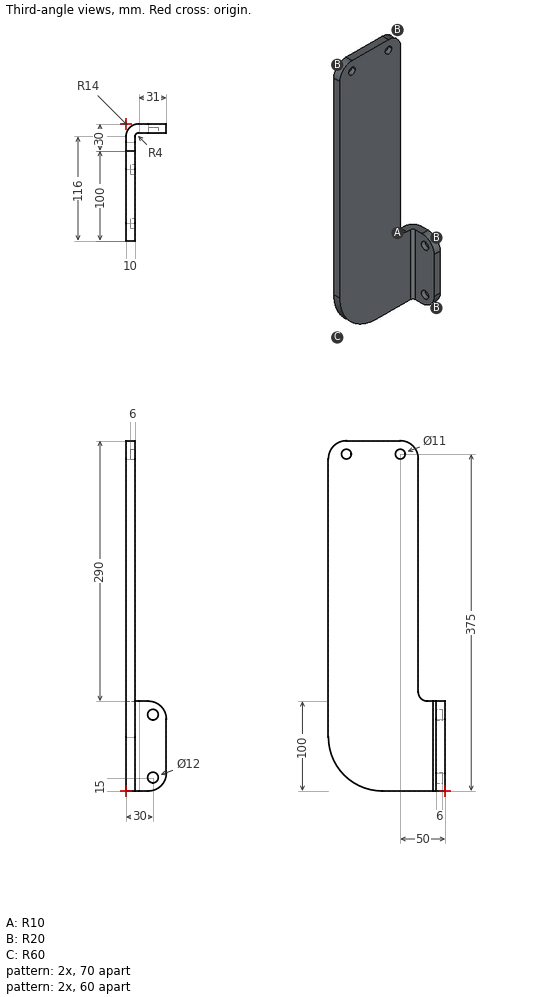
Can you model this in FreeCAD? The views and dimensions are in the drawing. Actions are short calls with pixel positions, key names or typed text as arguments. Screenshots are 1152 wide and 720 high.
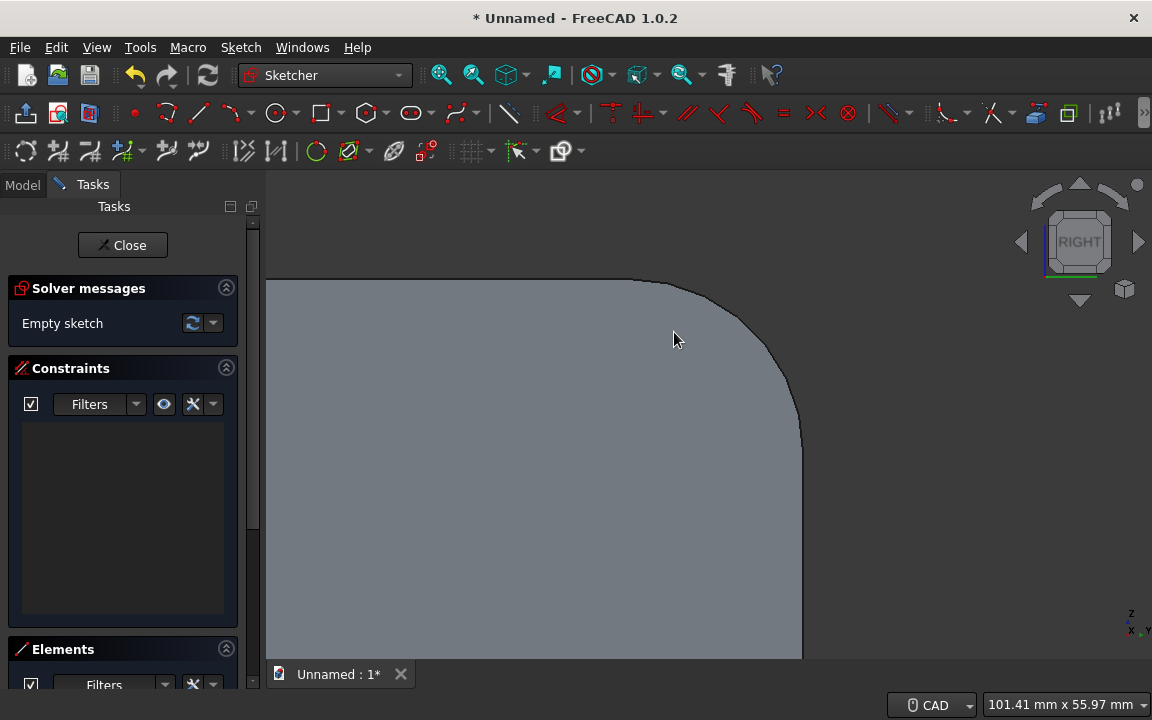
scroll(623, 408, up, 6)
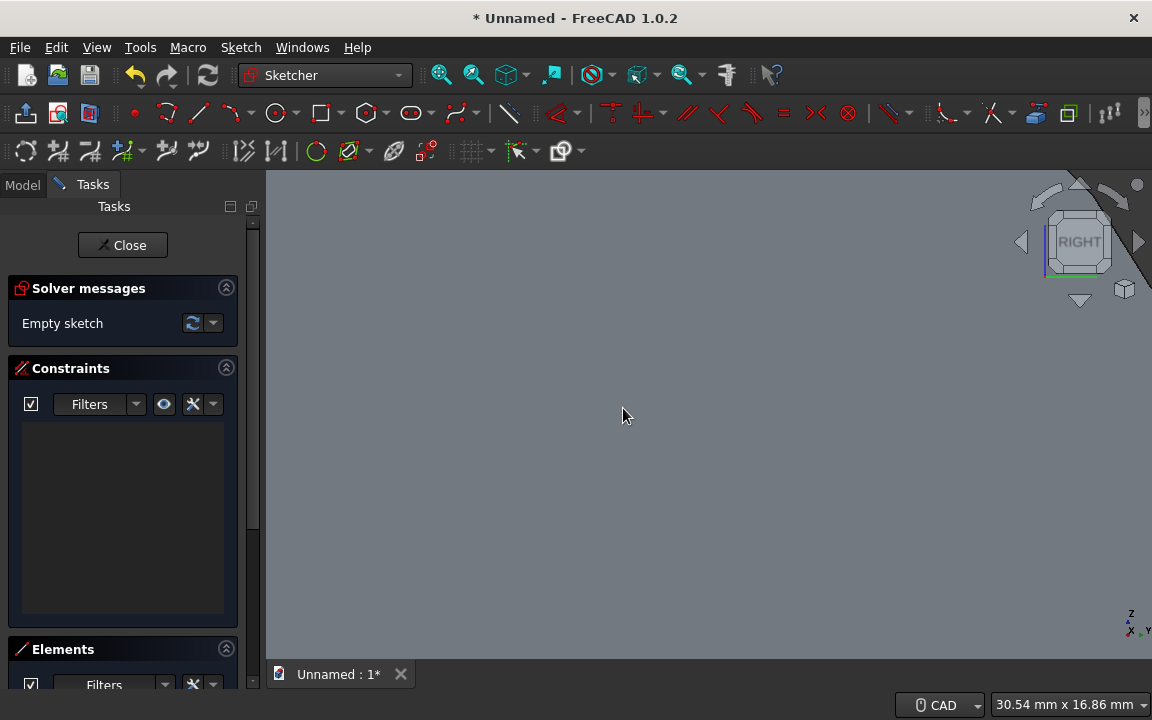
click(276, 114)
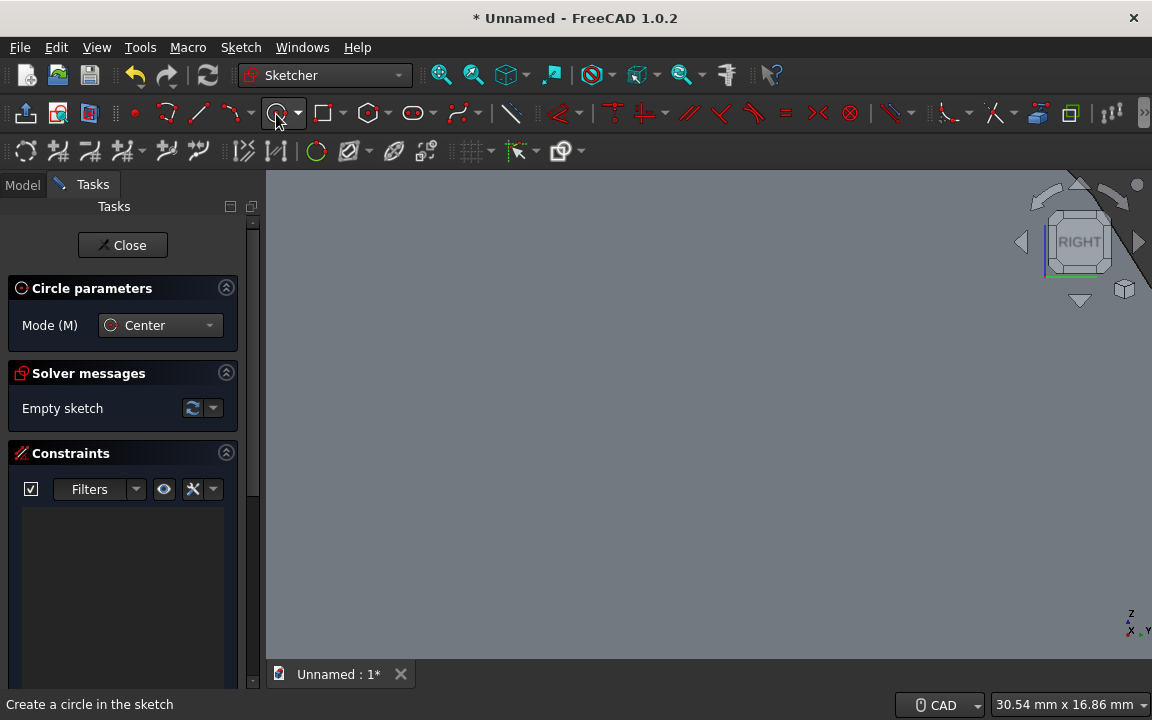
click(641, 414)
move(753, 301)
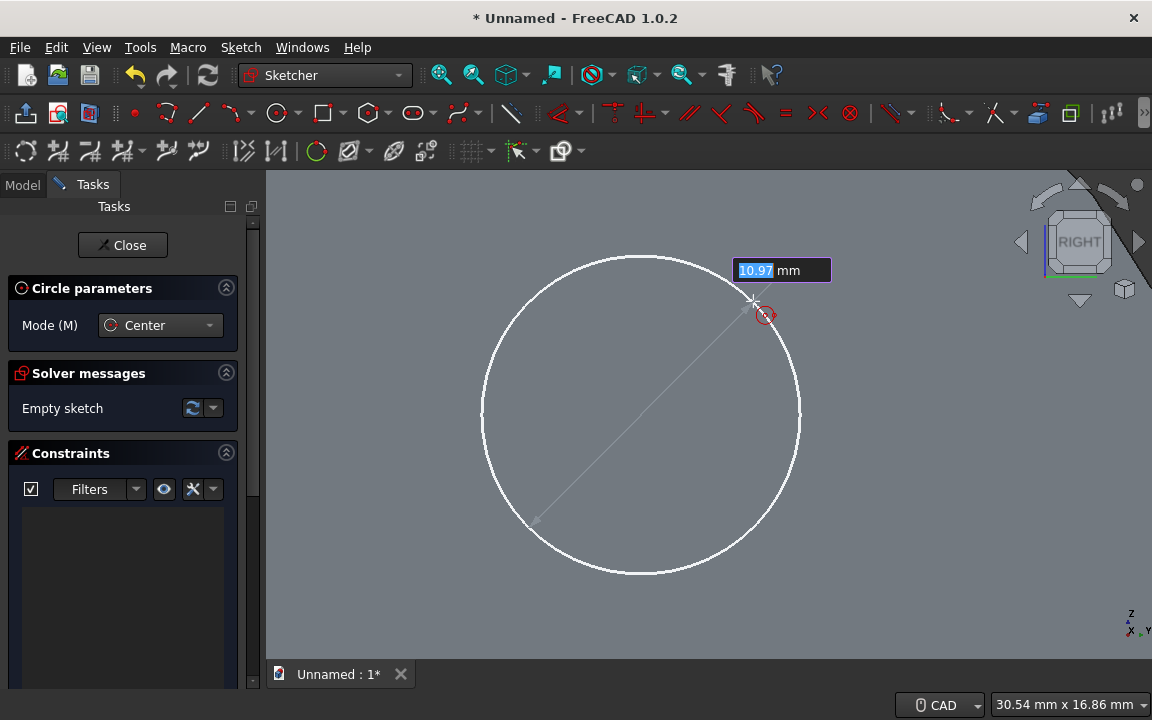
text(11)
key(Return)
key(Escape)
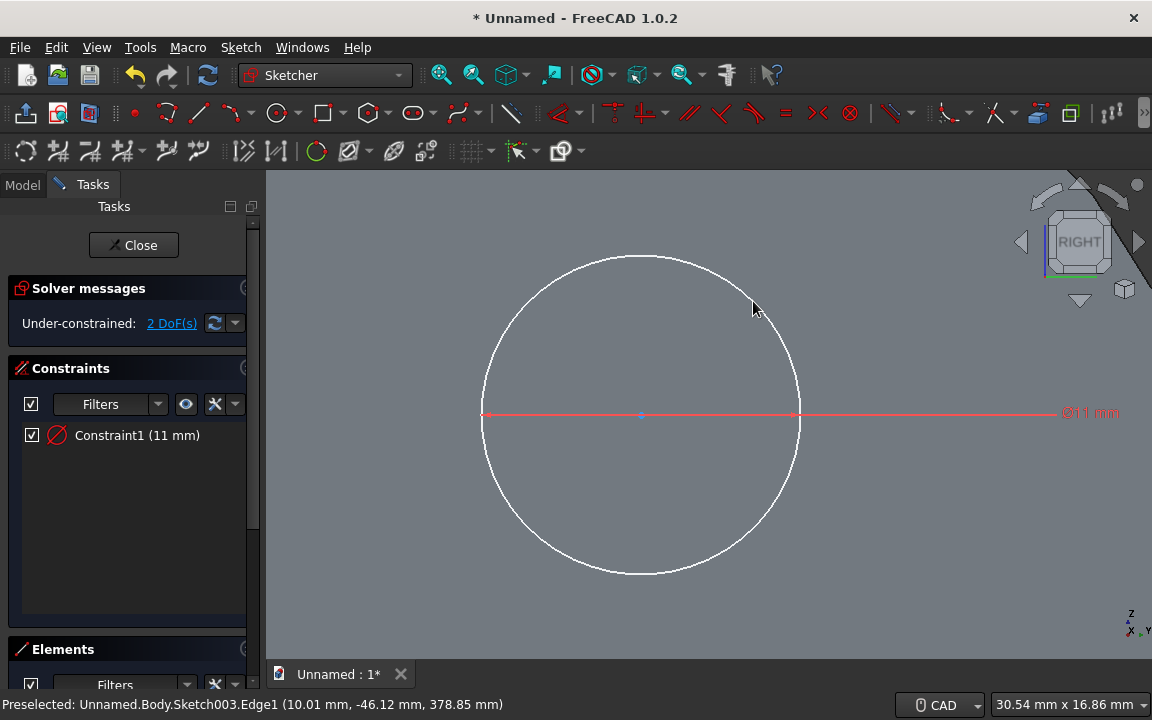
key(d)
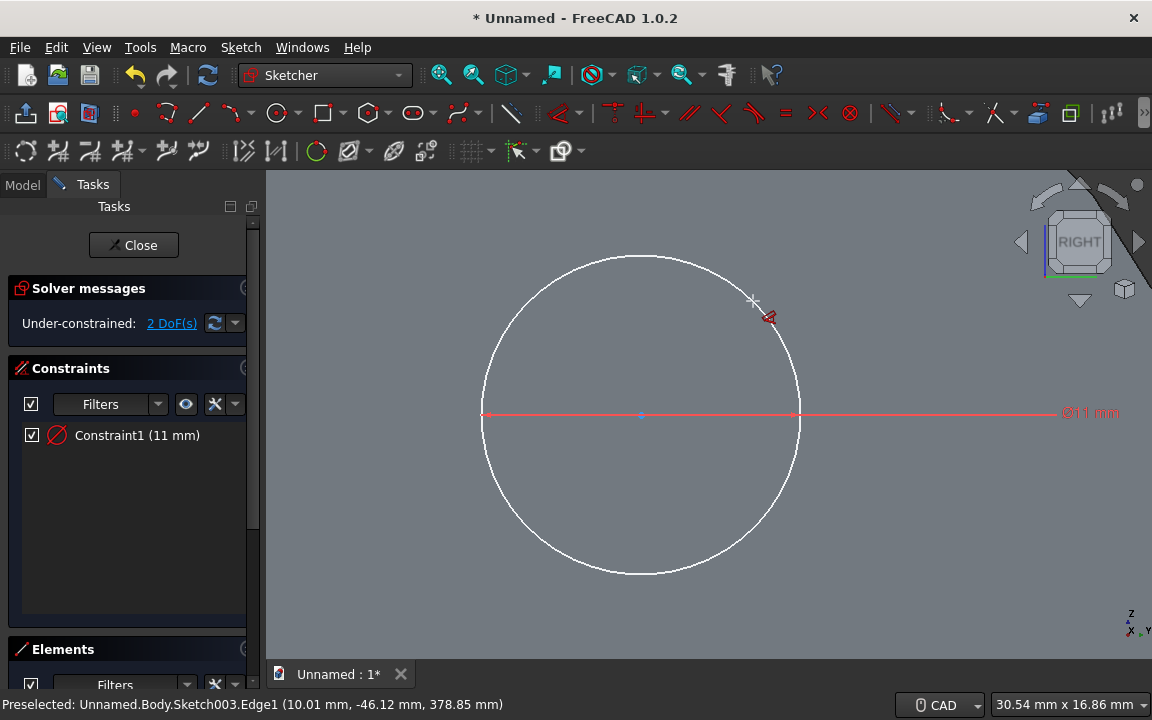
click(641, 415)
click(814, 381)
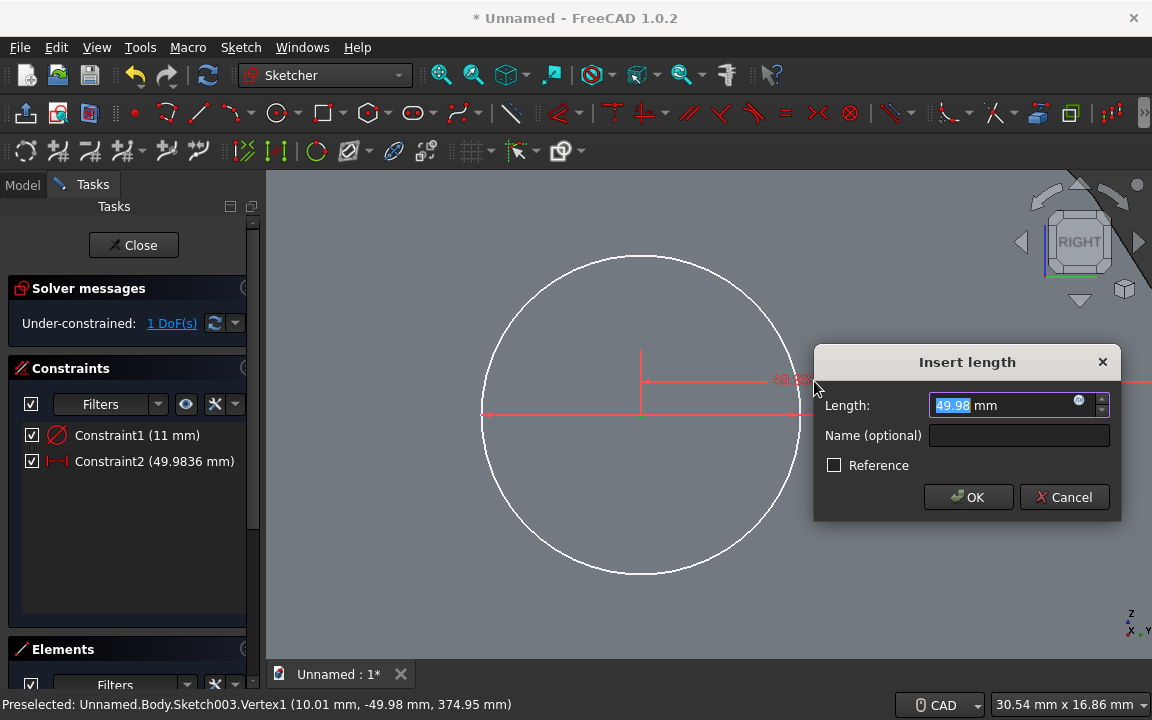
text(50)
key(Return)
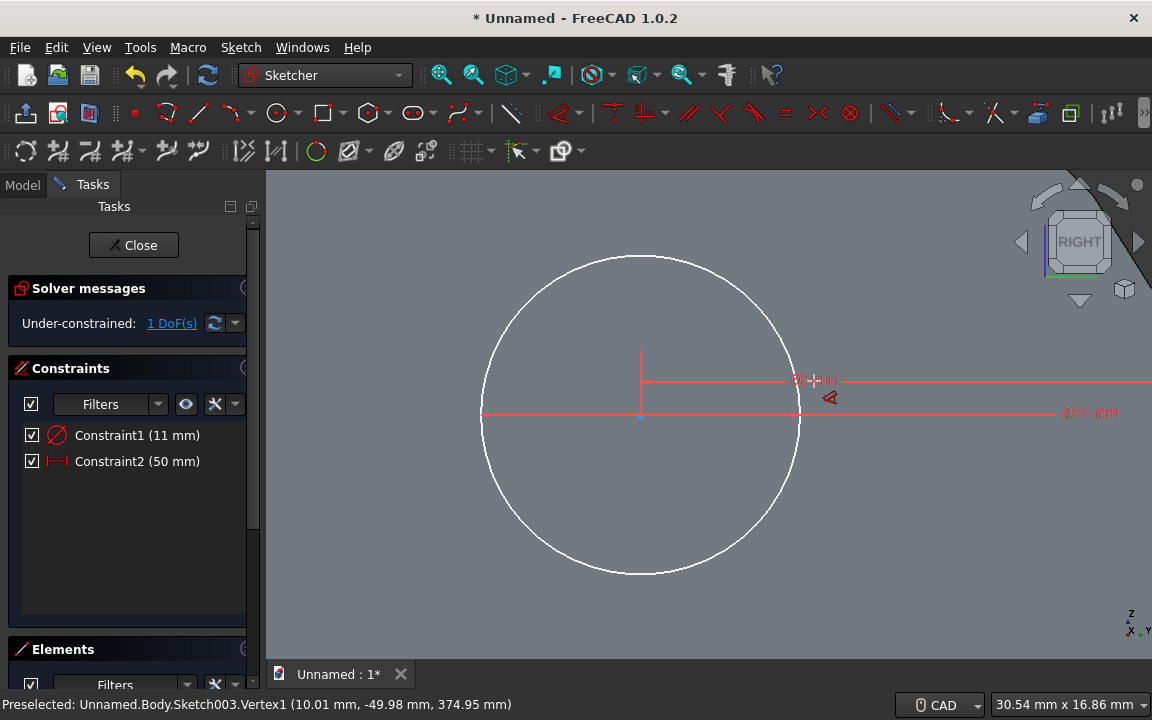
click(641, 415)
click(607, 523)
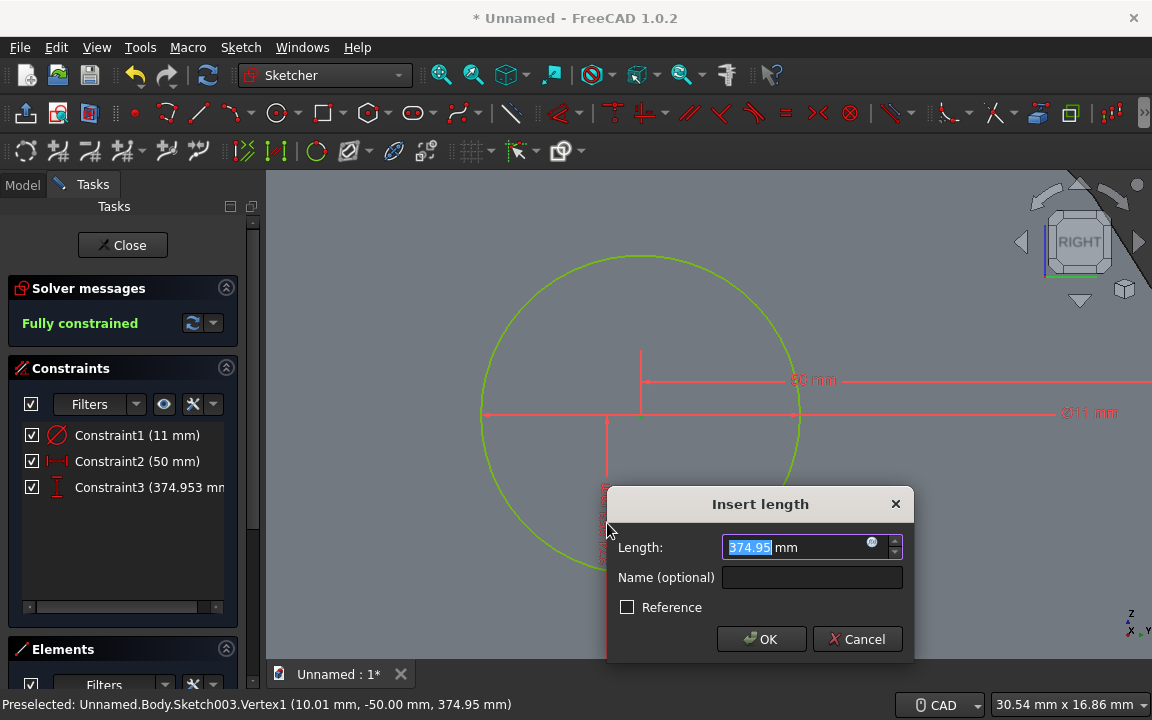
text(375)
key(Return)
key(Escape)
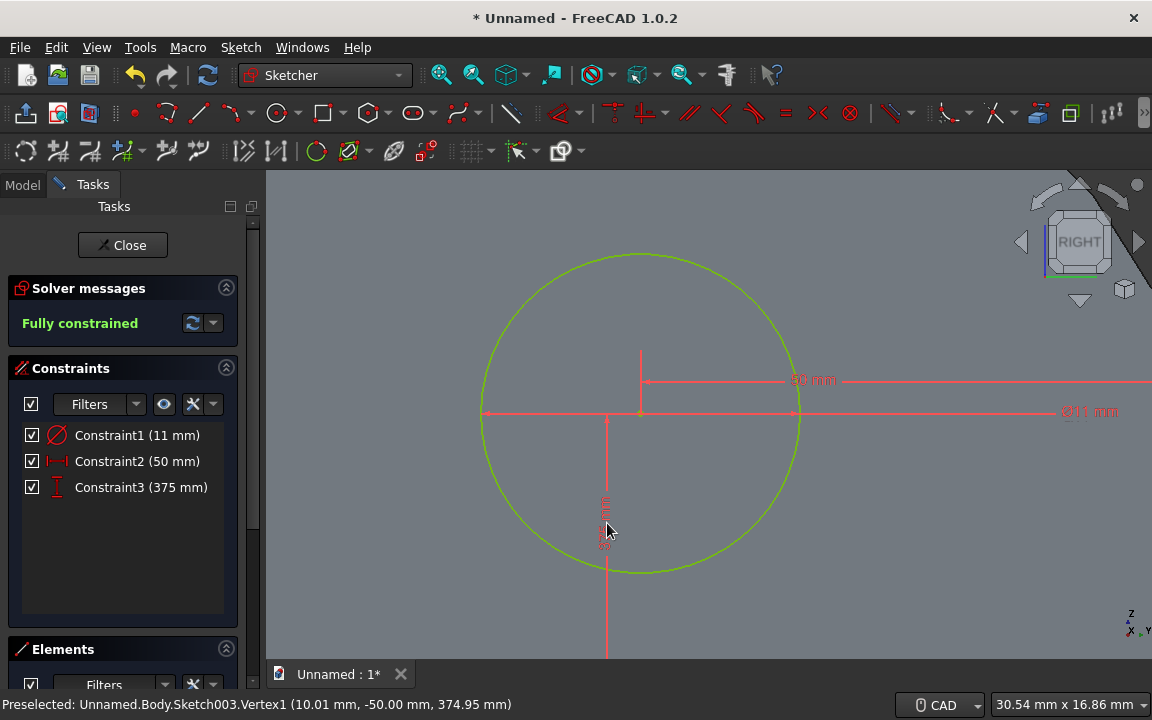
click(123, 245)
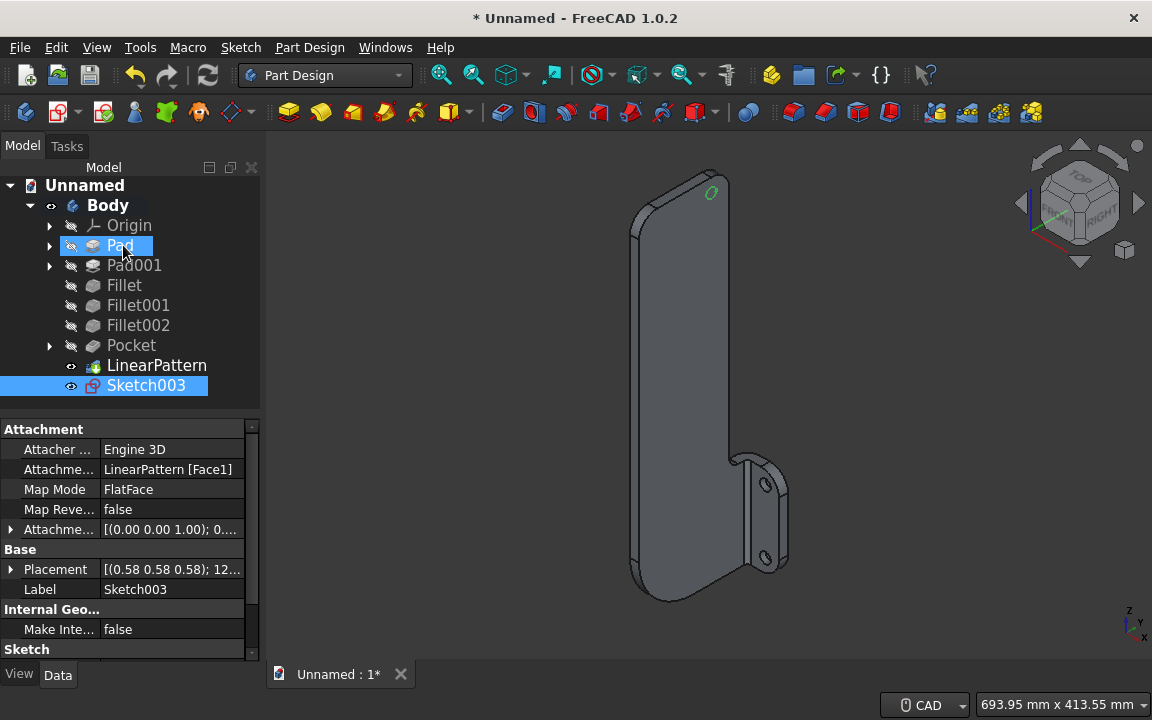
click(504, 112)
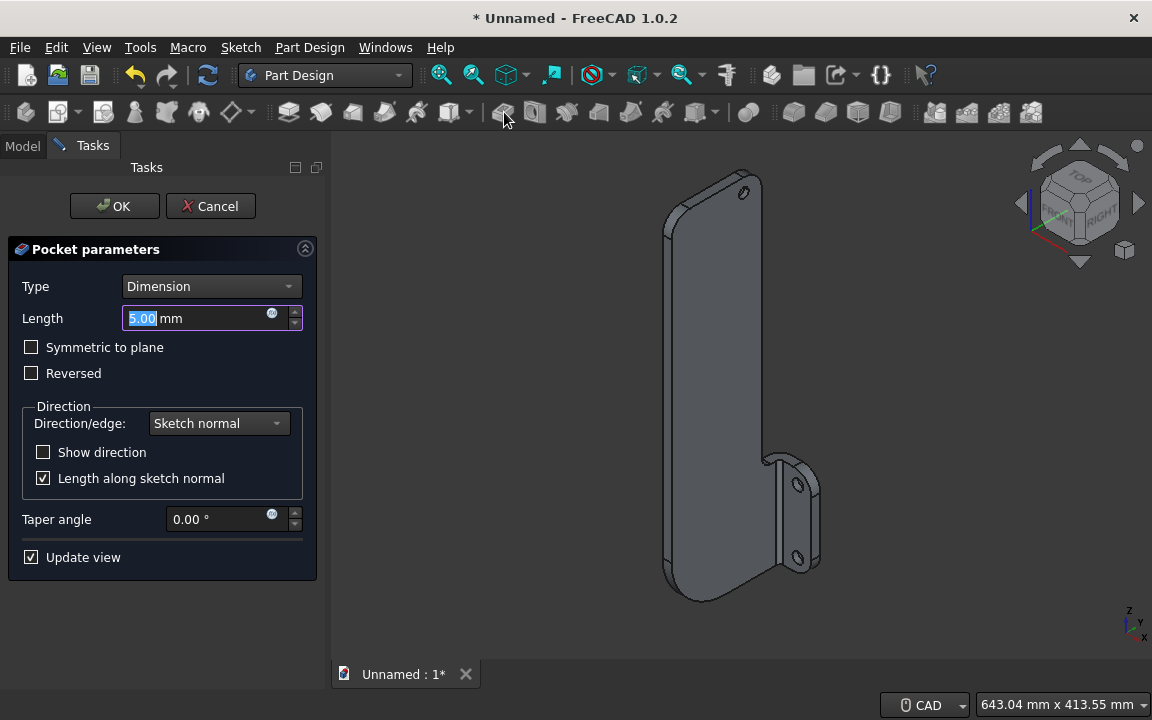
text(6)
key(Tab)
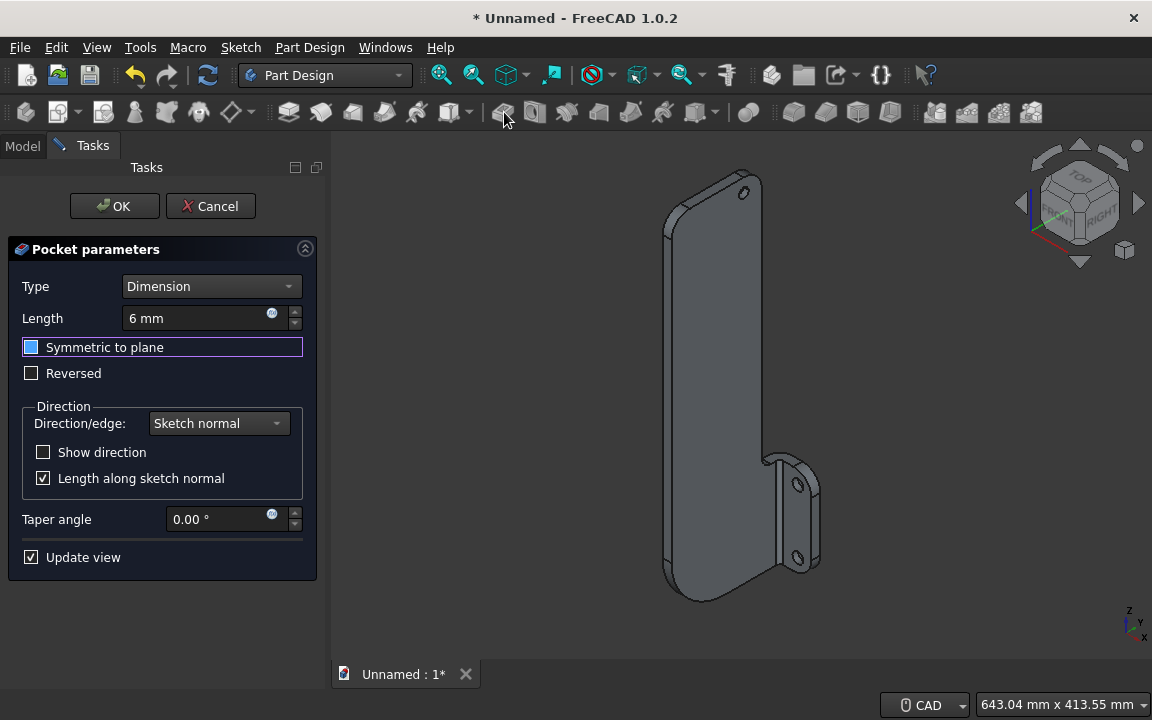
click(115, 206)